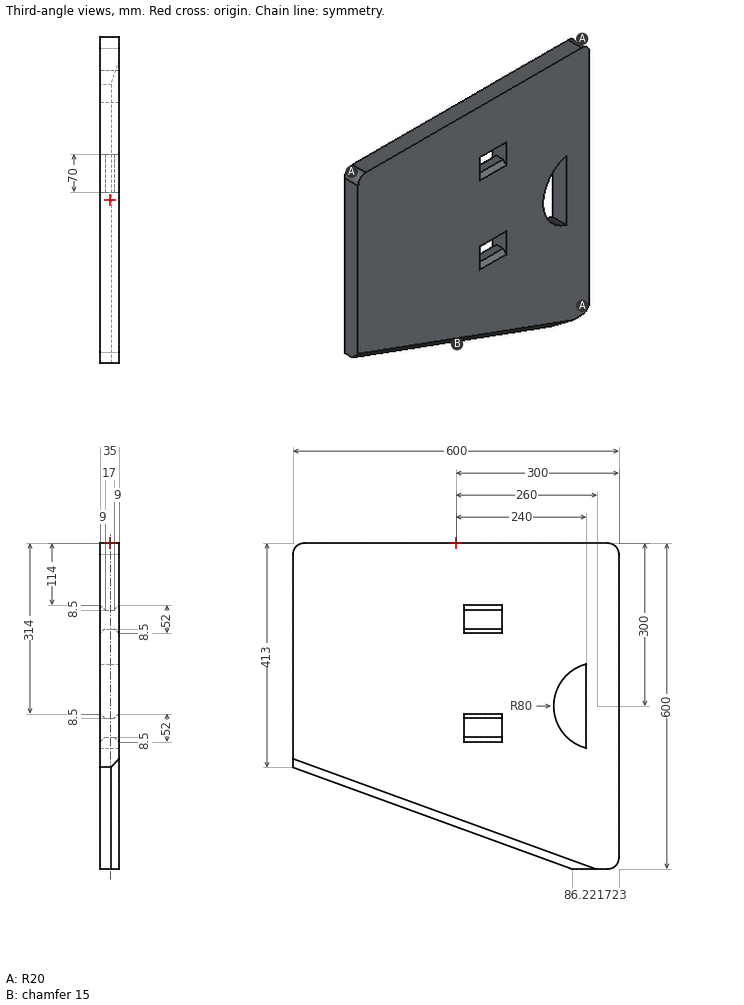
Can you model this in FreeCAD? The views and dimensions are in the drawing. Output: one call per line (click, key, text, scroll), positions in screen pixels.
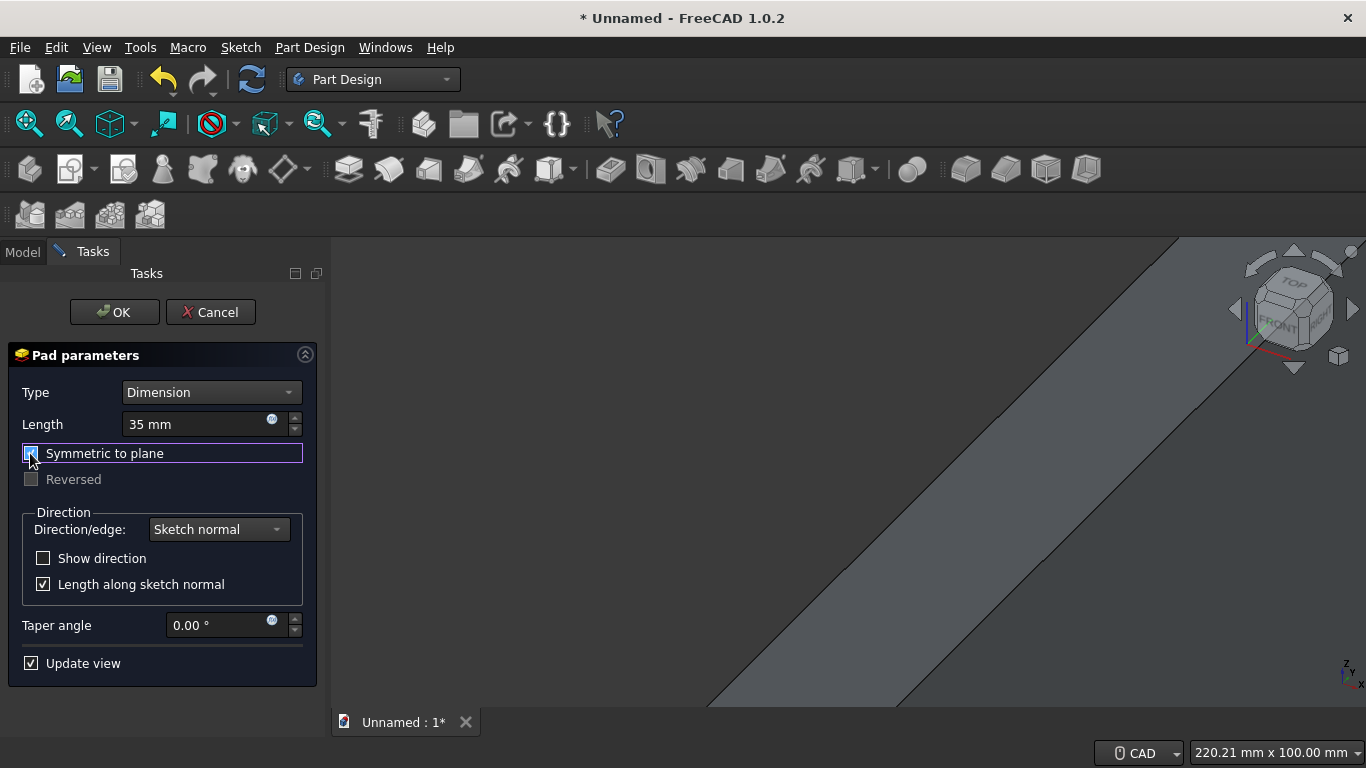
click(115, 312)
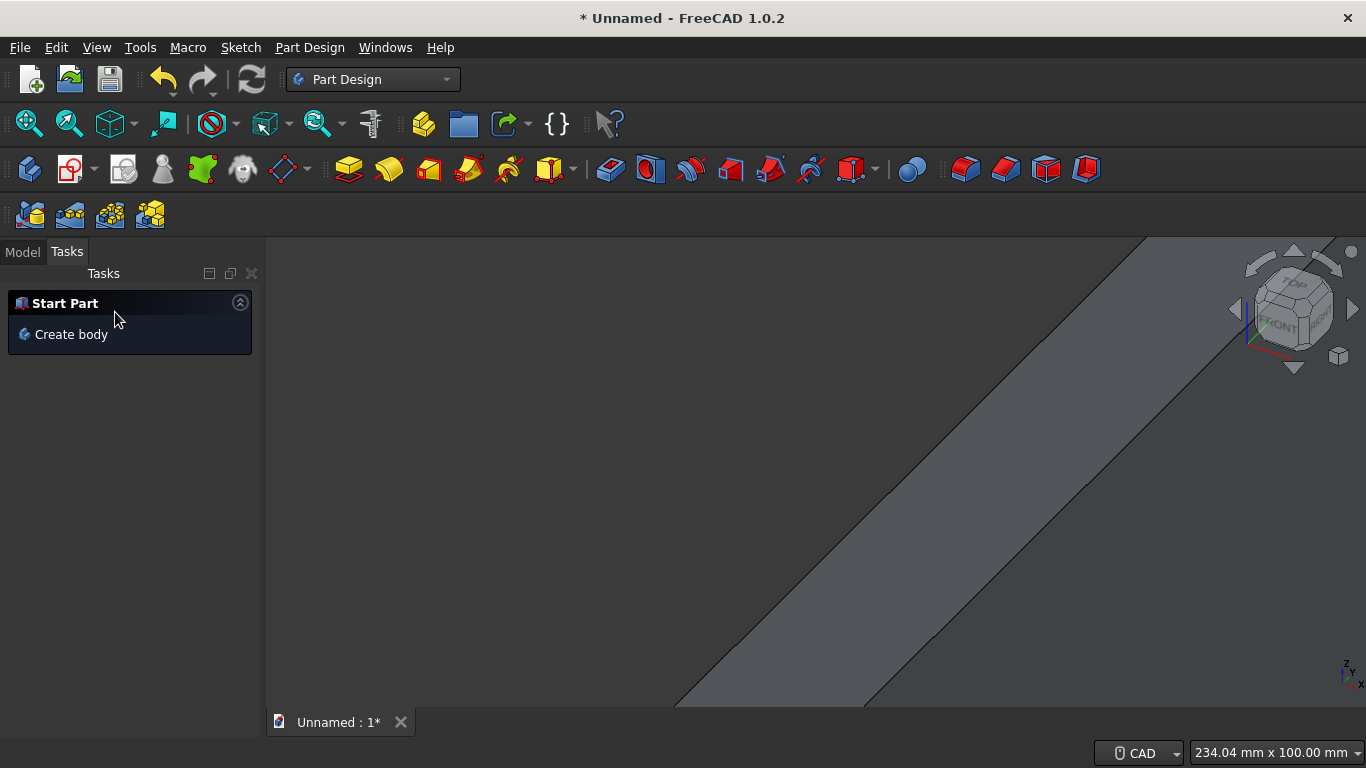
key(v)
key(f)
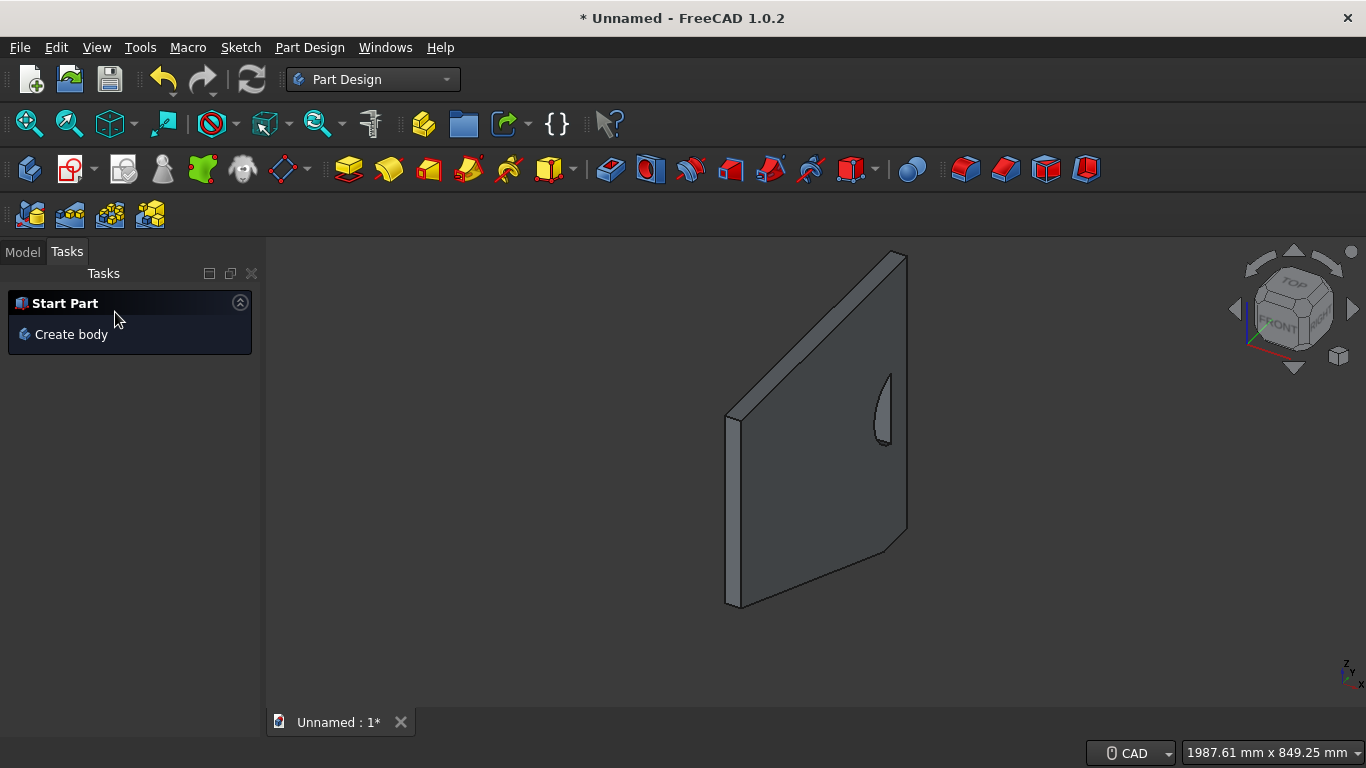
click(23, 251)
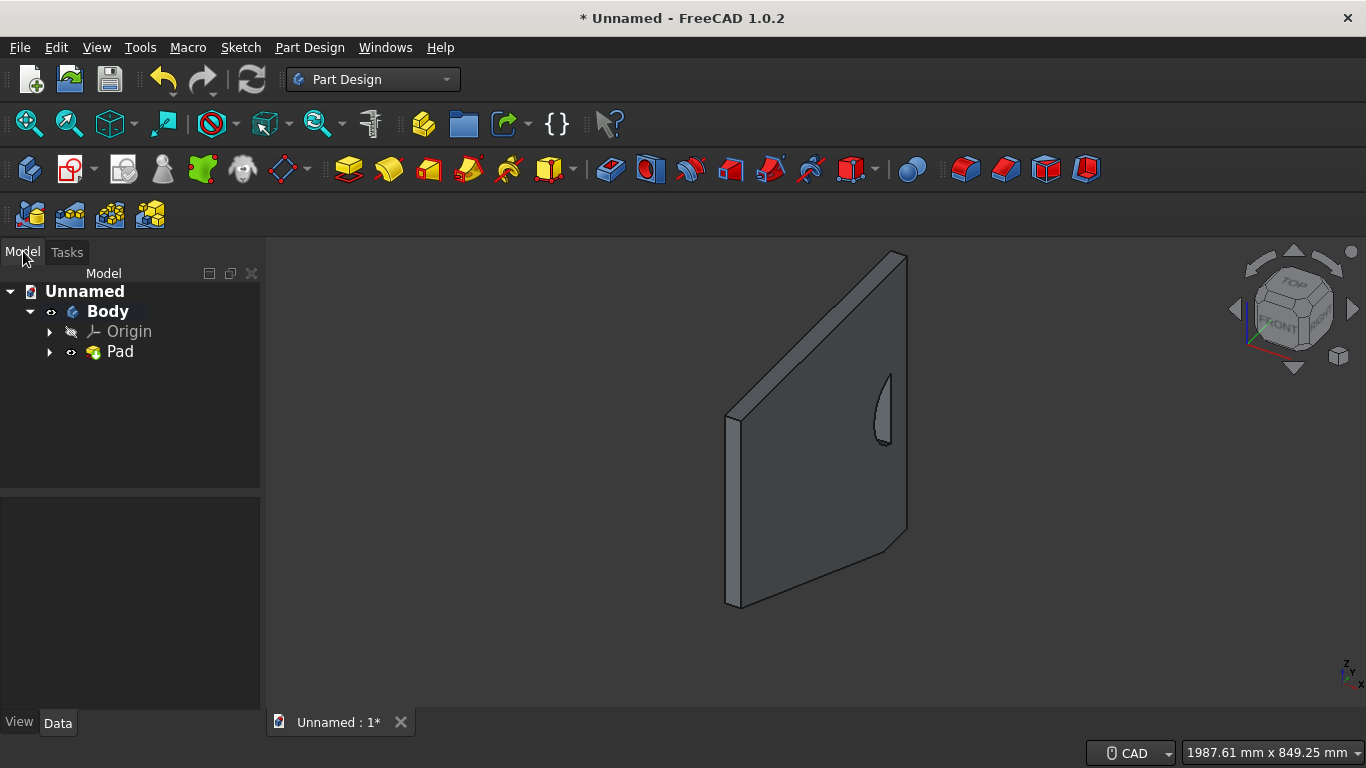
click(50, 332)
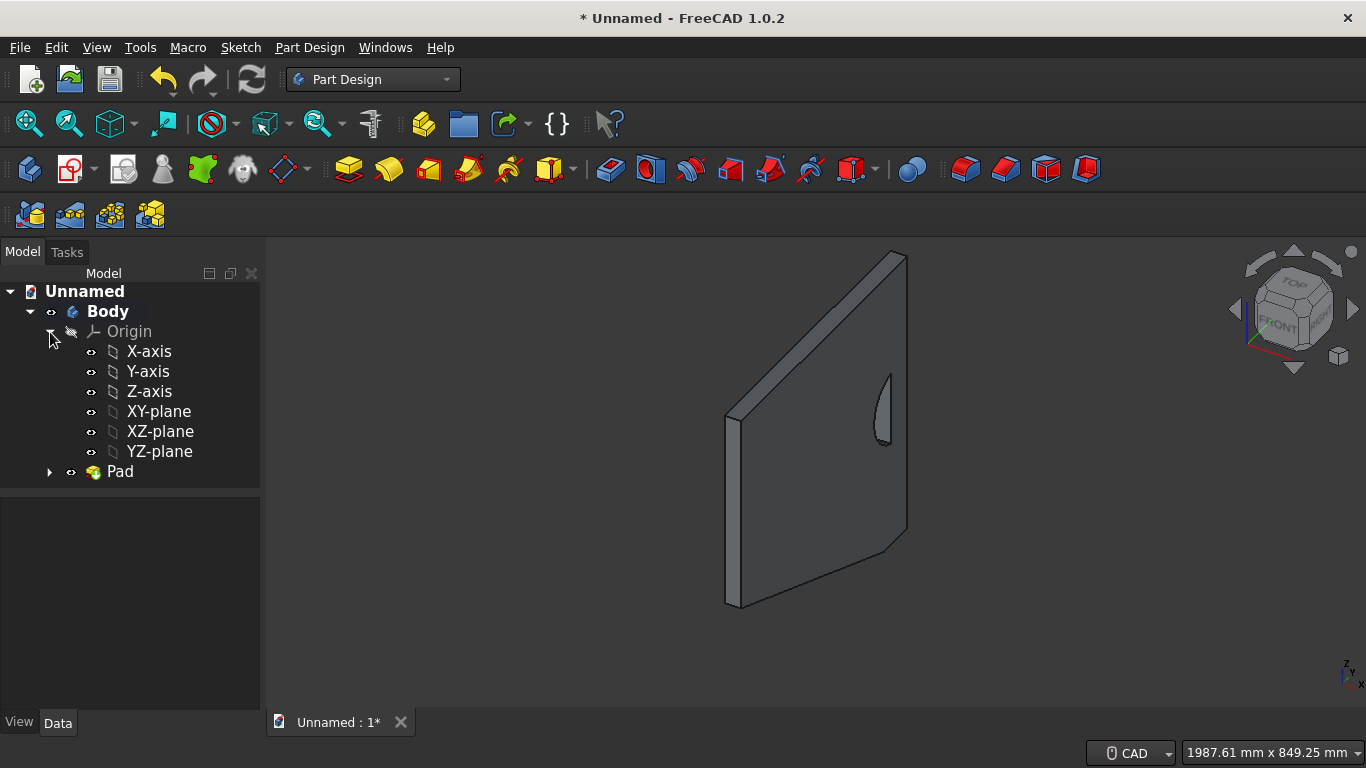
click(136, 432)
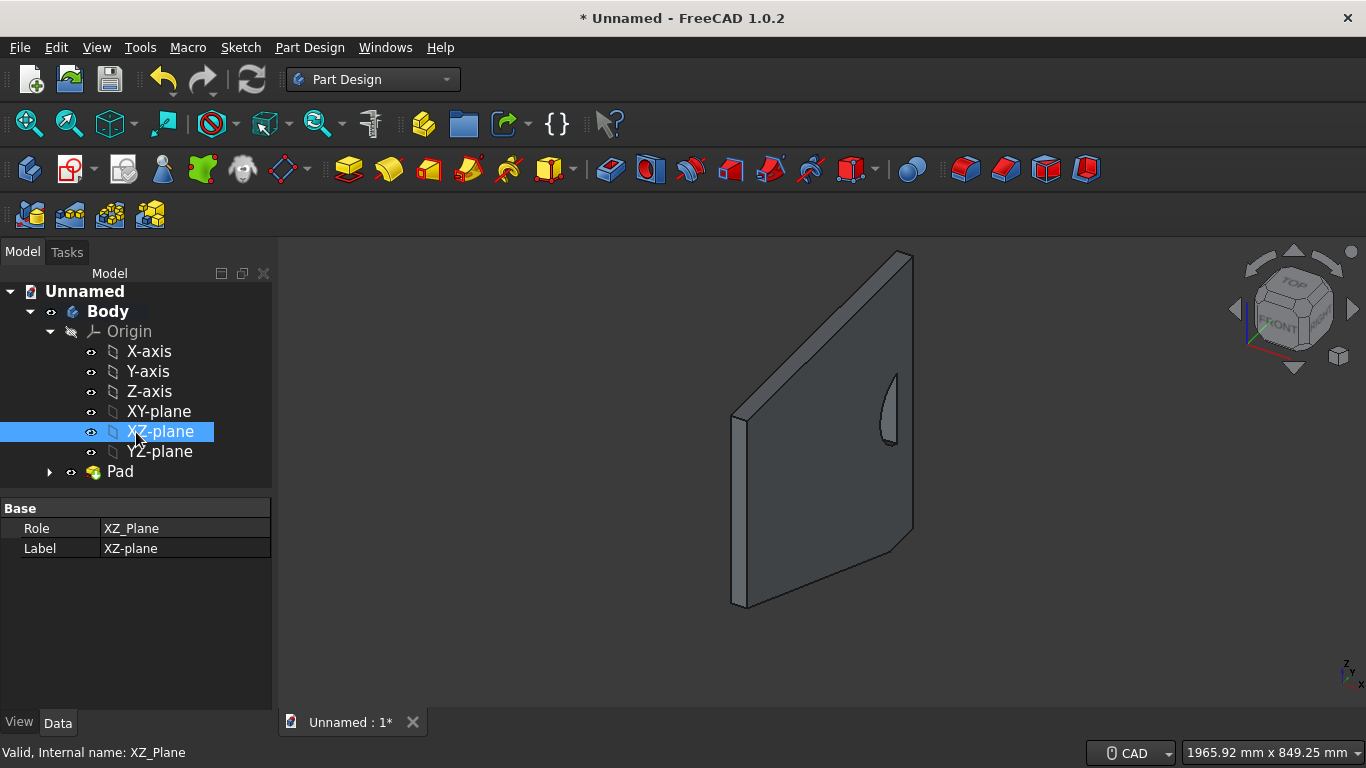
click(284, 170)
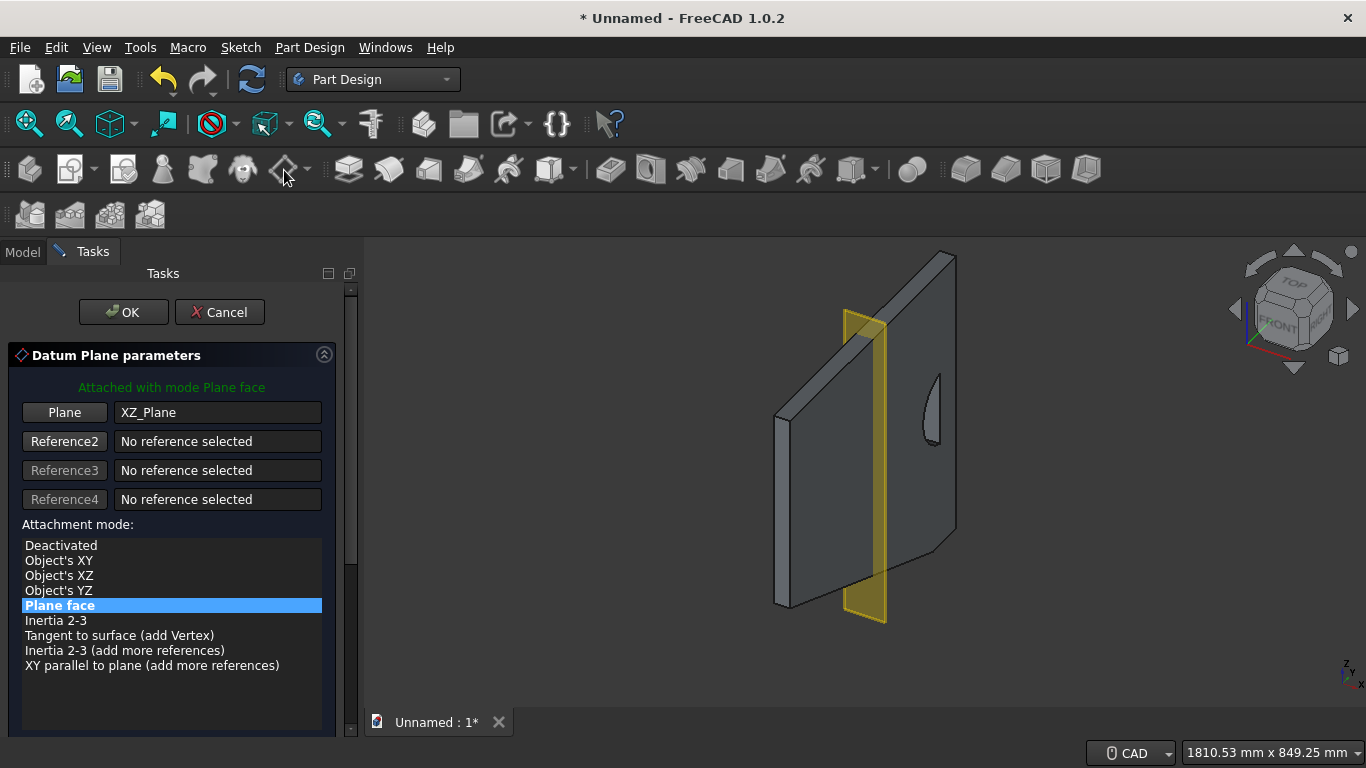
scroll(351, 510, down, 3)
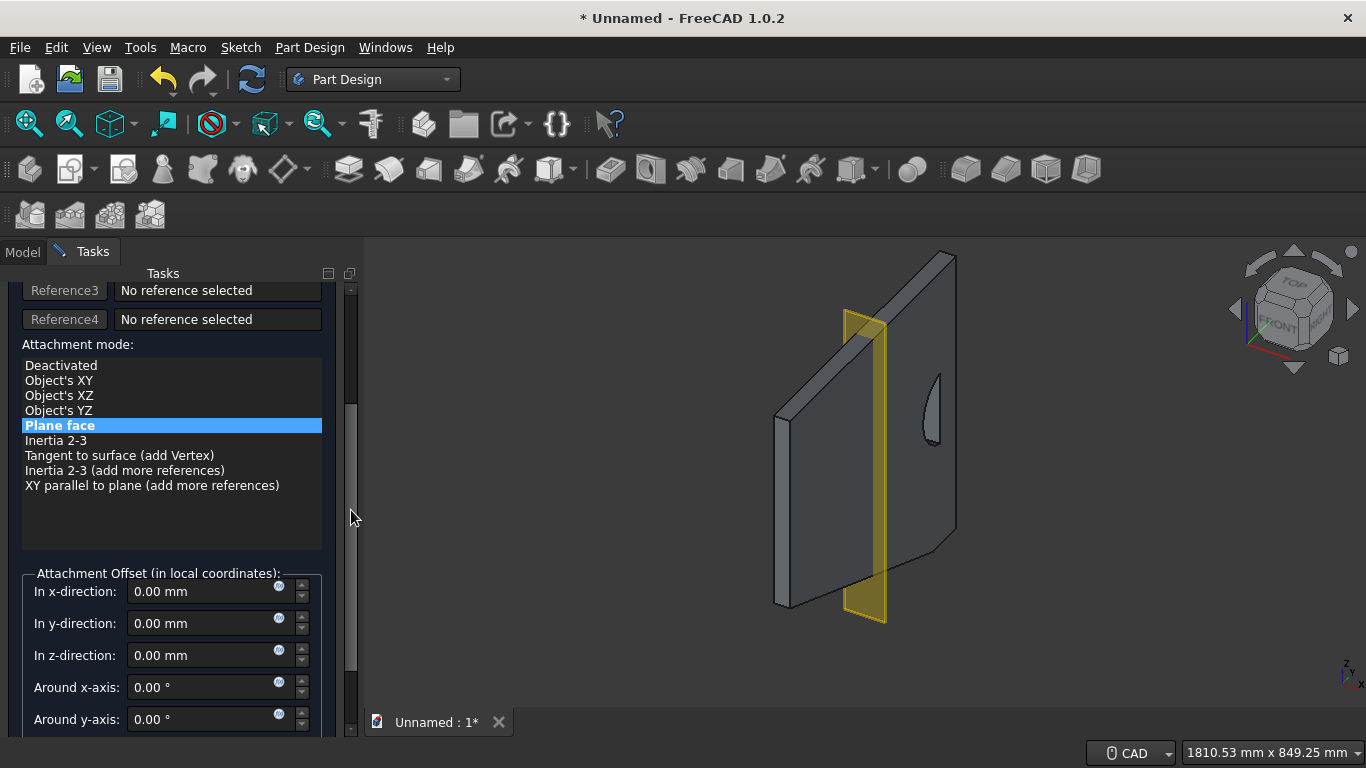
triple_click(210, 655)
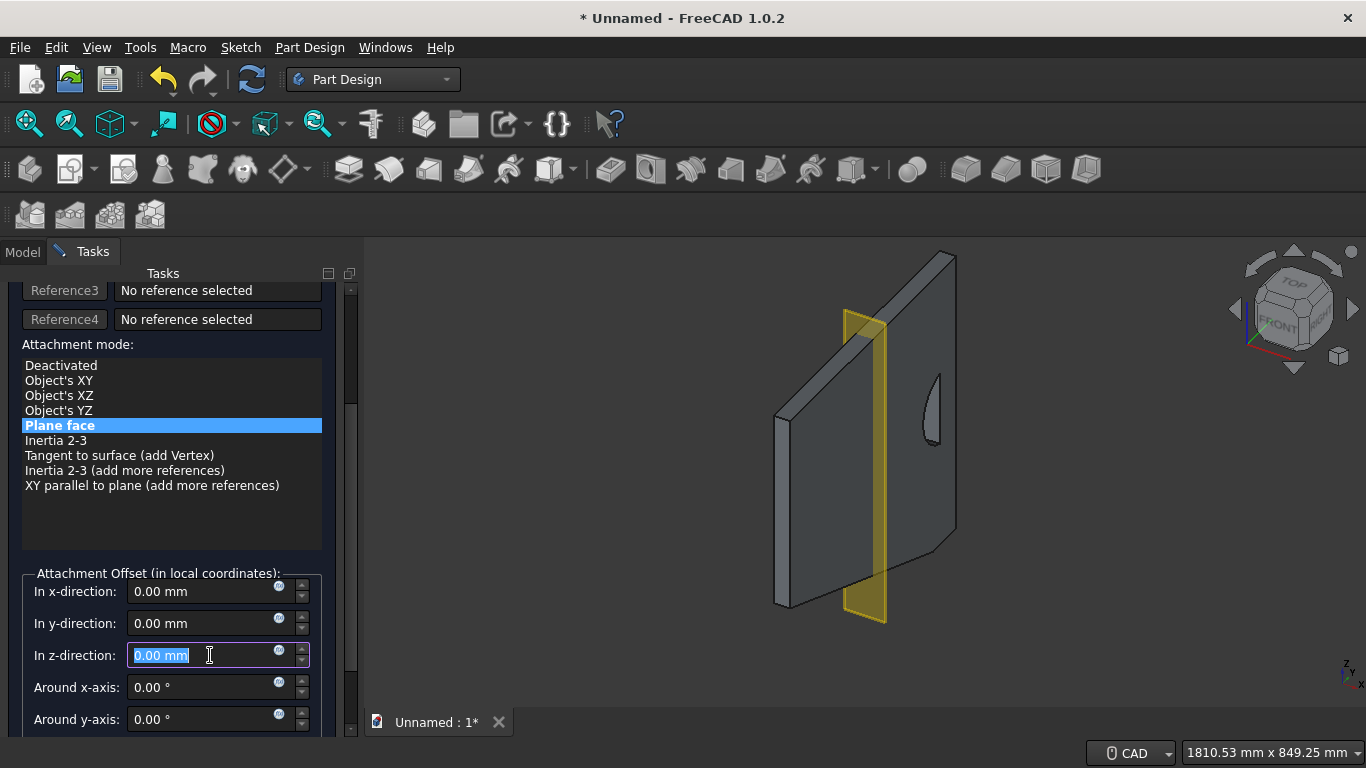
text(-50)
key(Tab)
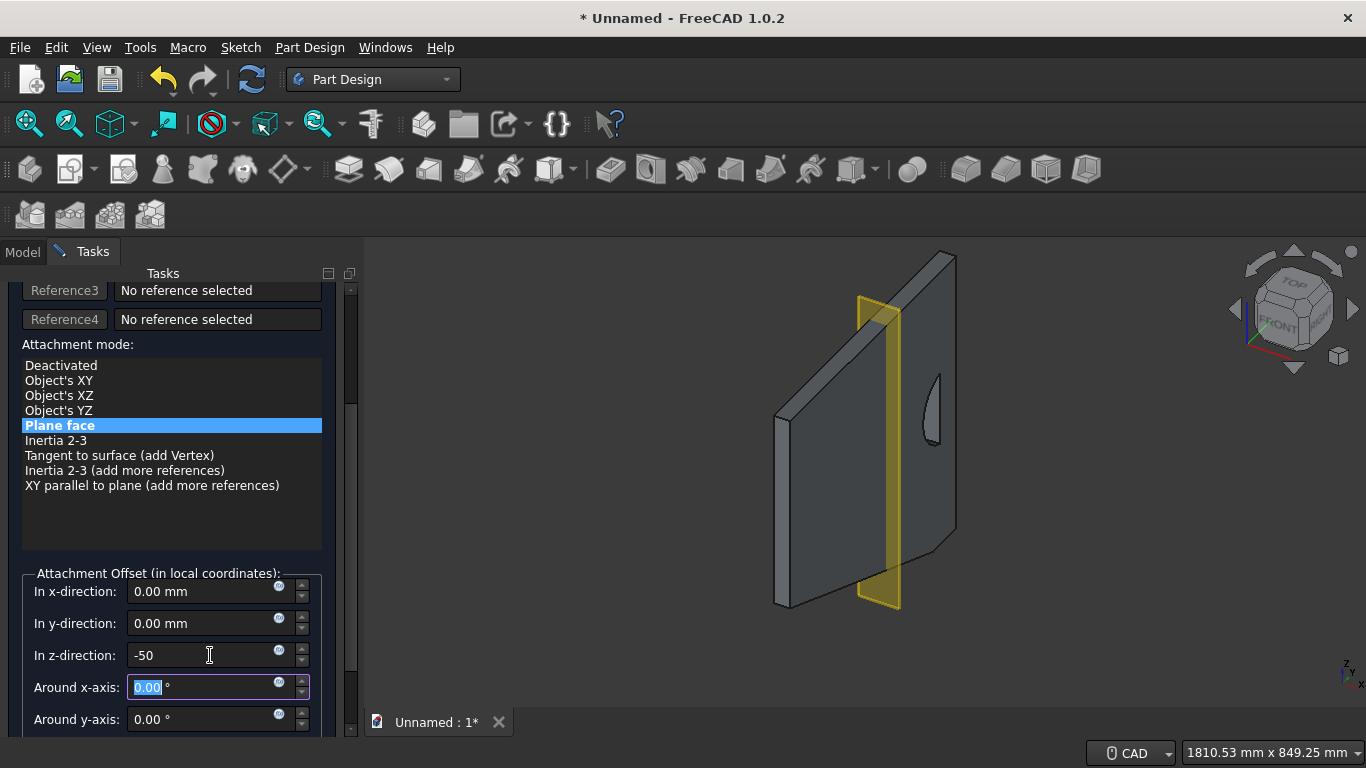
scroll(351, 510, up, 4)